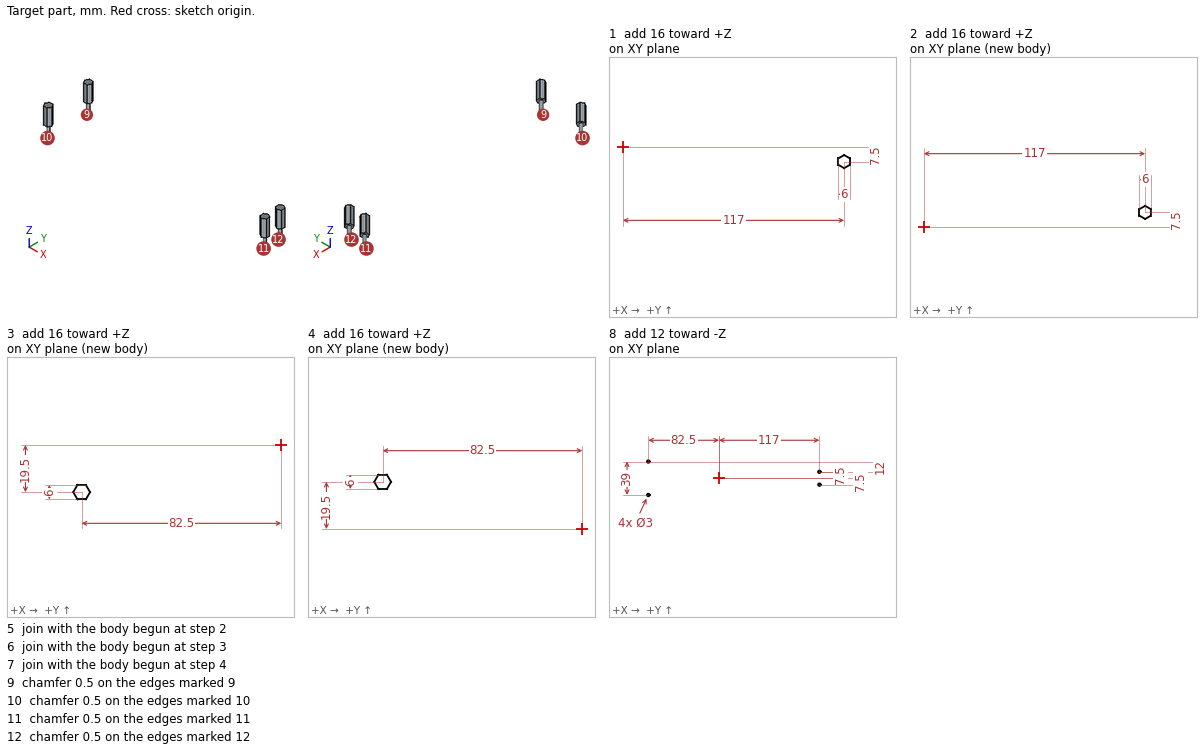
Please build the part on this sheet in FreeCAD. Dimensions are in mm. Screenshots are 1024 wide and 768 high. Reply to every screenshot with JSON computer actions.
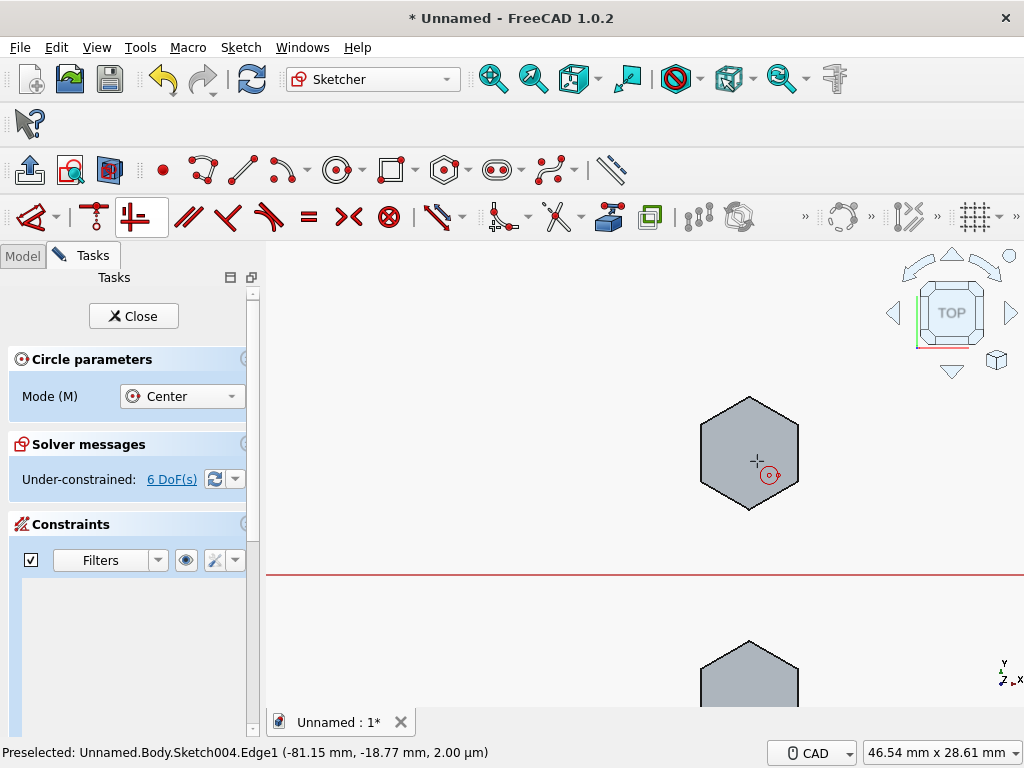
{"action": "scroll", "coordinate": [757, 461], "scroll_direction": "down", "scroll_amount": 11}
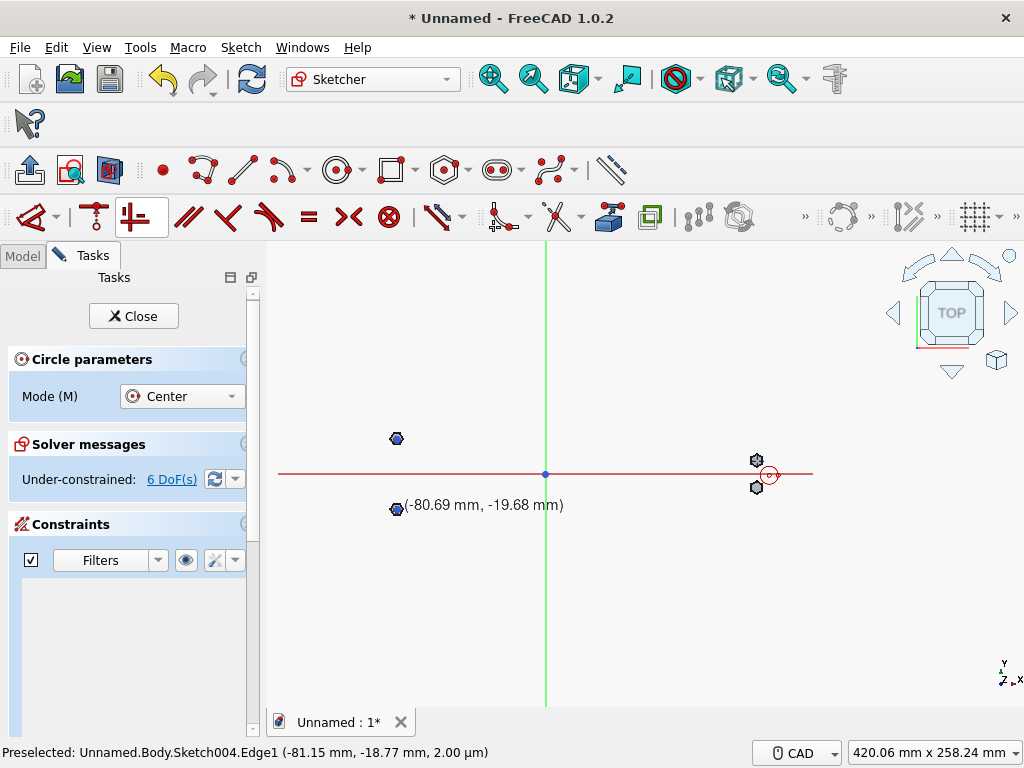
{"action": "left_click", "coordinate": [757, 461]}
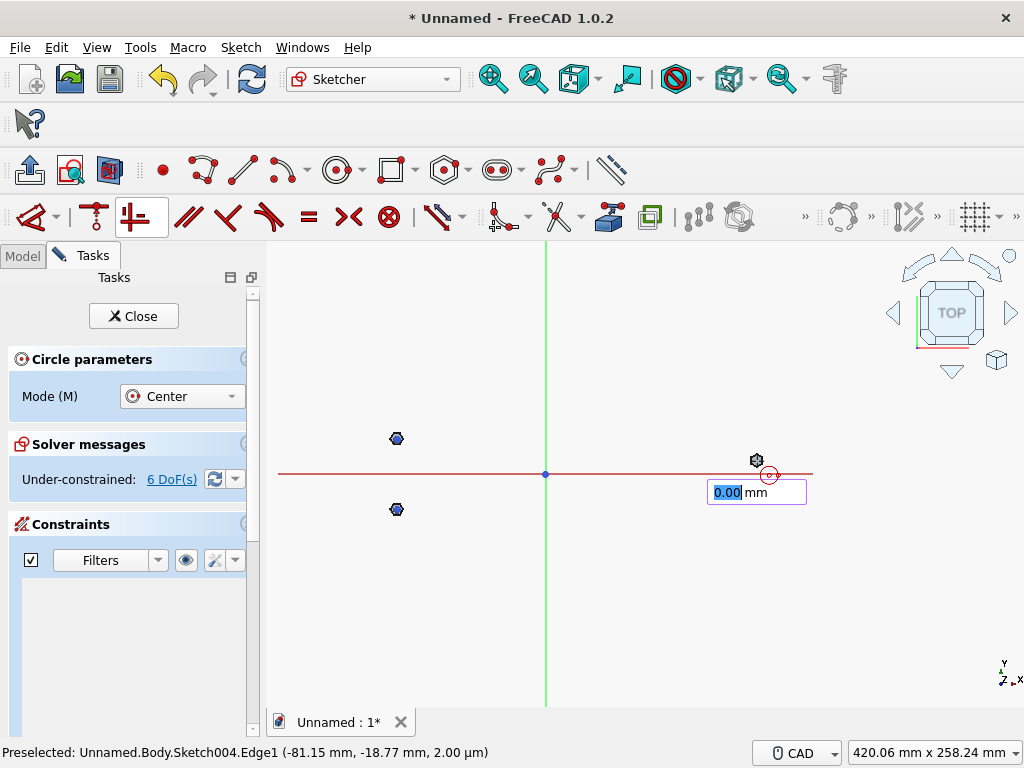
{"action": "scroll", "coordinate": [759, 459], "scroll_direction": "up", "scroll_amount": 9}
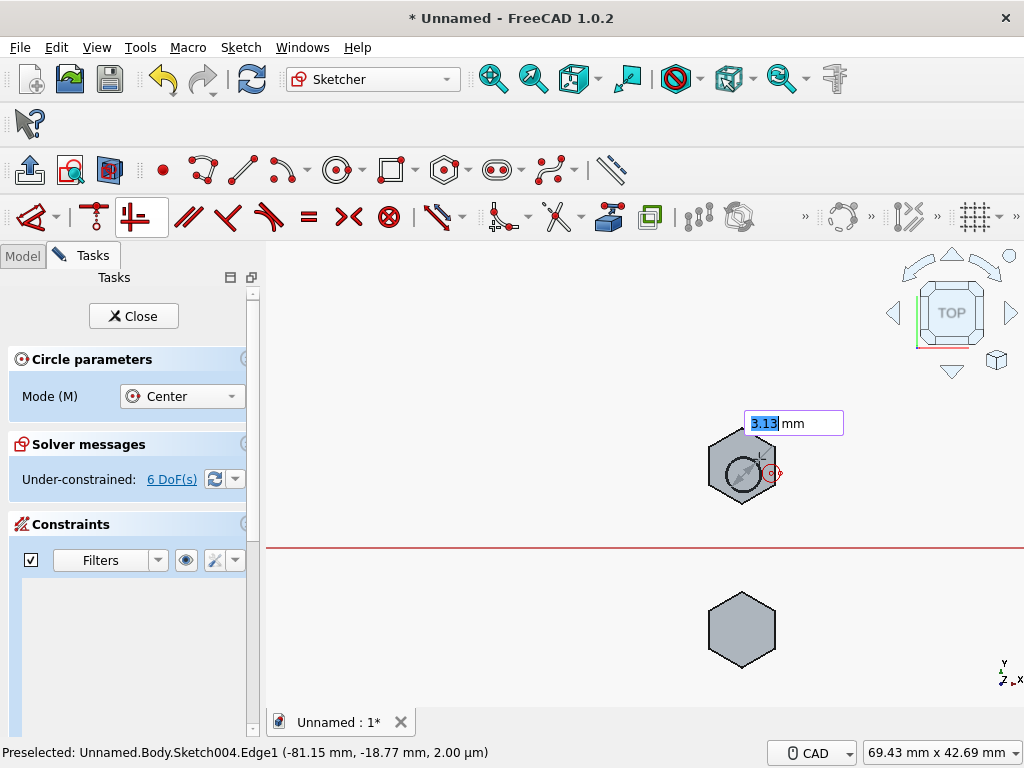
{"action": "left_click", "coordinate": [754, 454]}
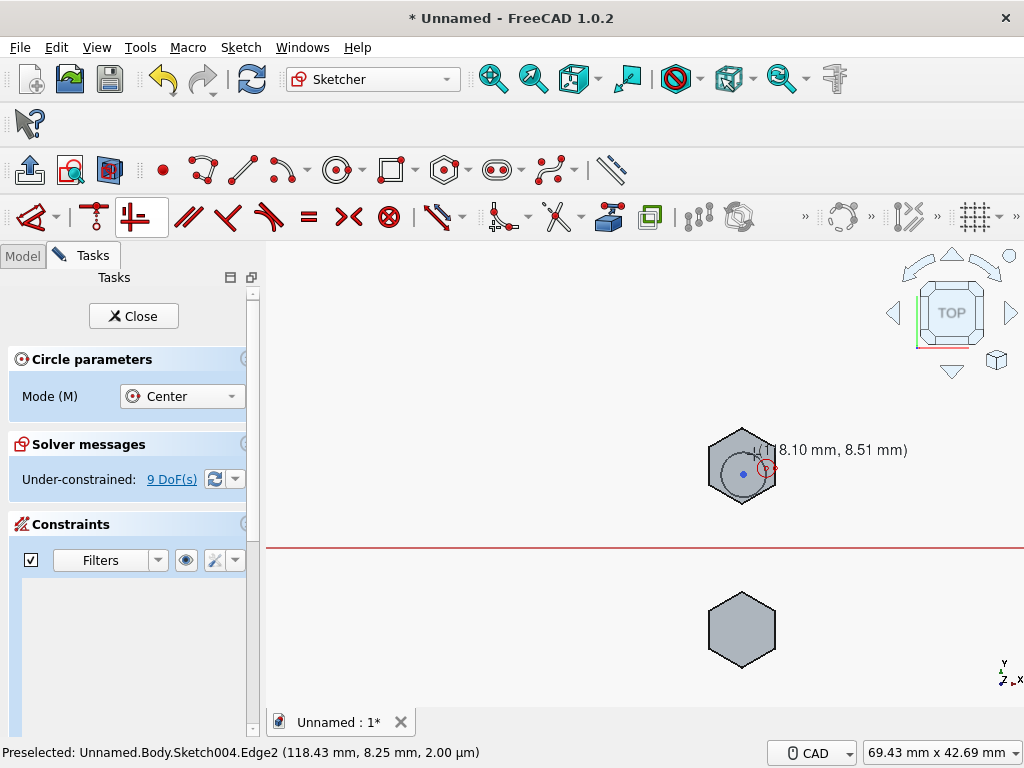
{"action": "scroll", "coordinate": [742, 630], "scroll_direction": "up", "scroll_amount": 2}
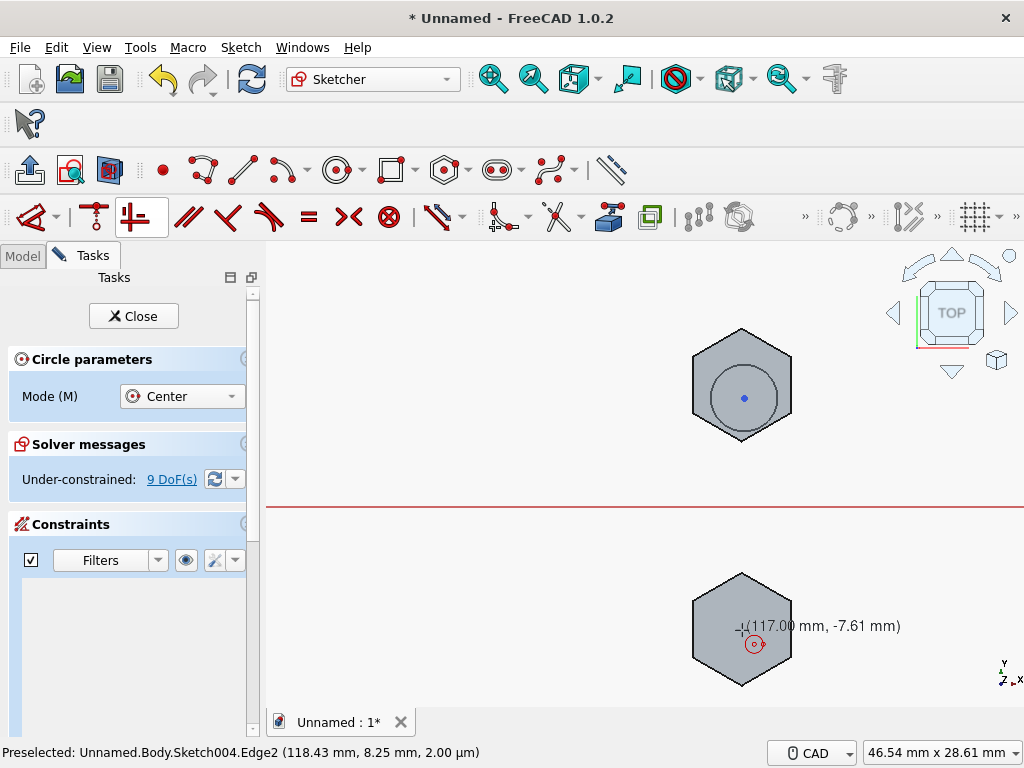
{"action": "scroll", "coordinate": [758, 470], "scroll_direction": "down", "scroll_amount": 11}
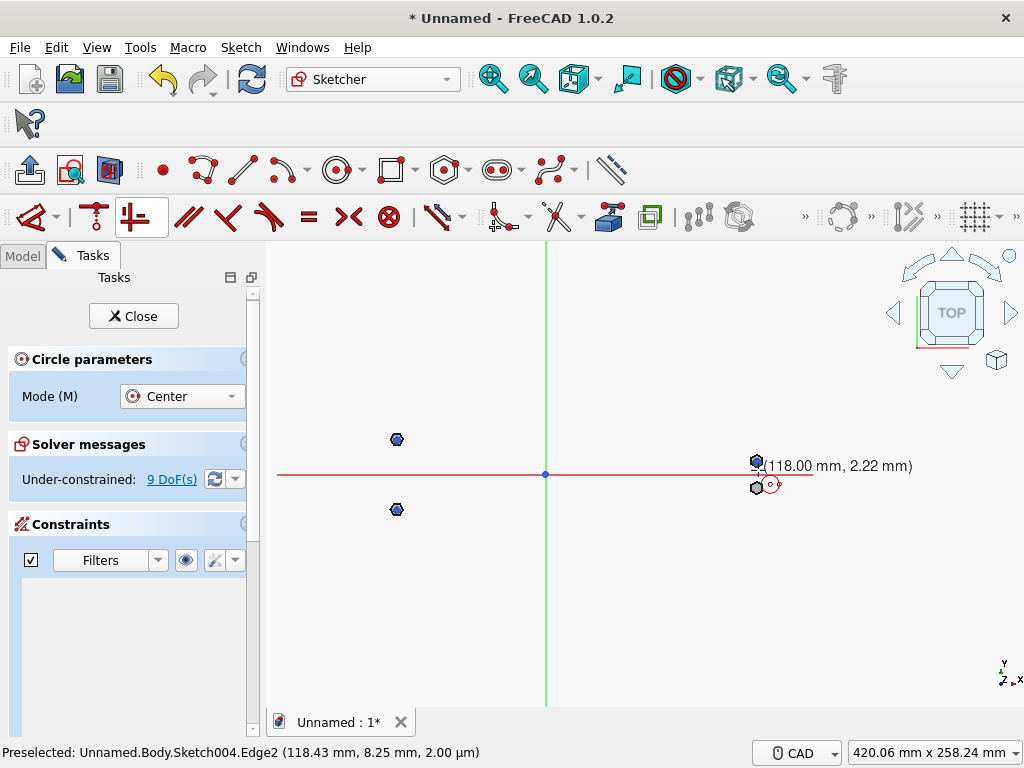
{"action": "left_click", "coordinate": [757, 488]}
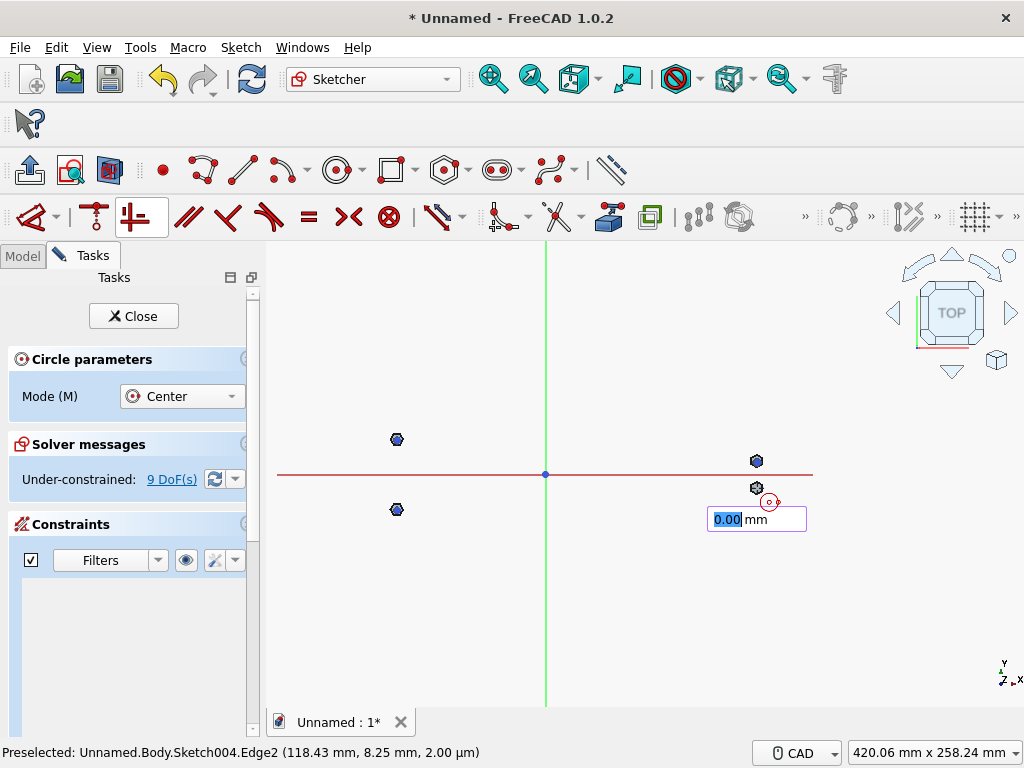
{"action": "scroll", "coordinate": [759, 490], "scroll_direction": "up", "scroll_amount": 9}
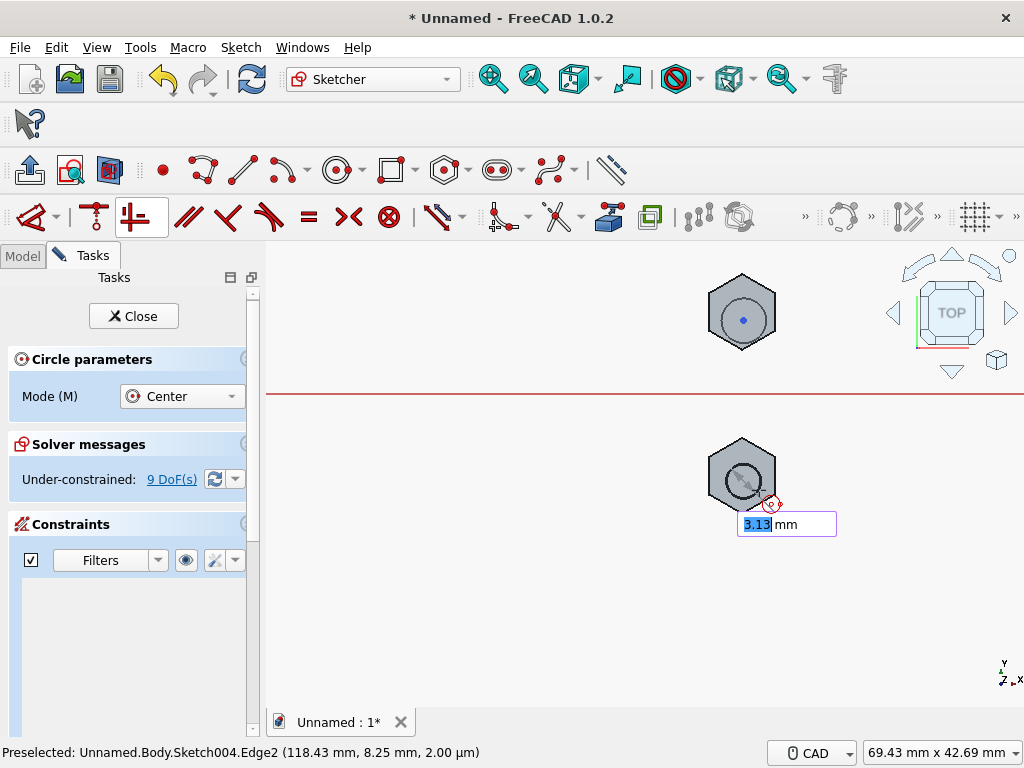
{"action": "left_click", "coordinate": [754, 487]}
{"action": "key", "text": "Escape"}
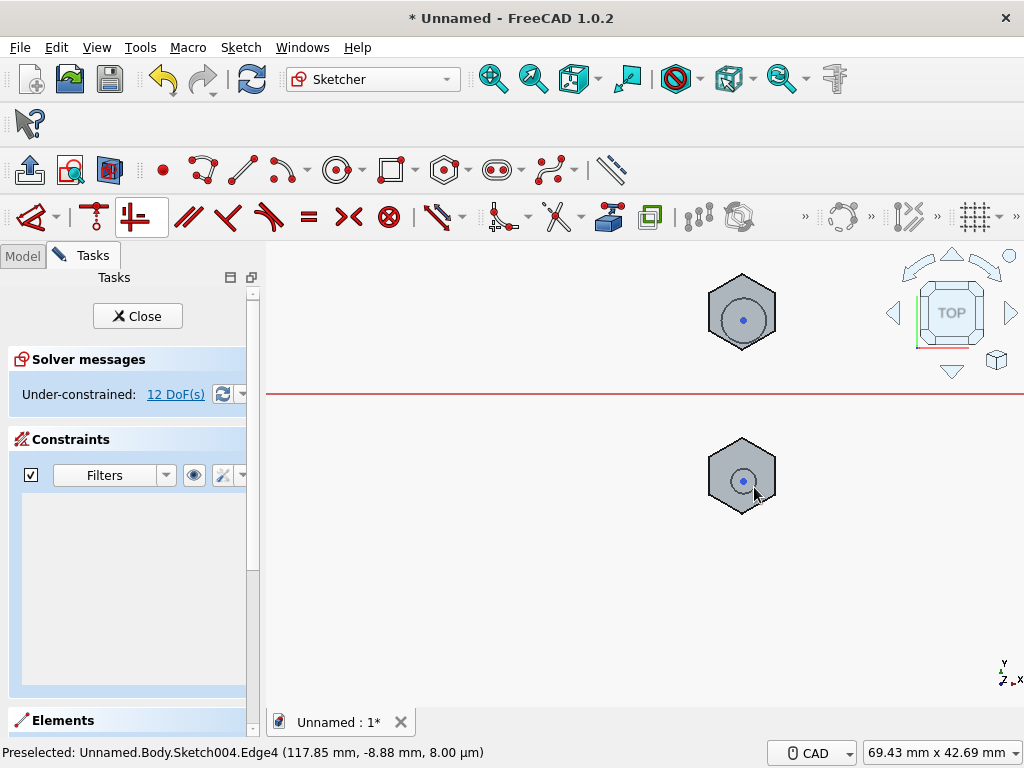
{"action": "scroll", "coordinate": [759, 490], "scroll_direction": "down", "scroll_amount": 9}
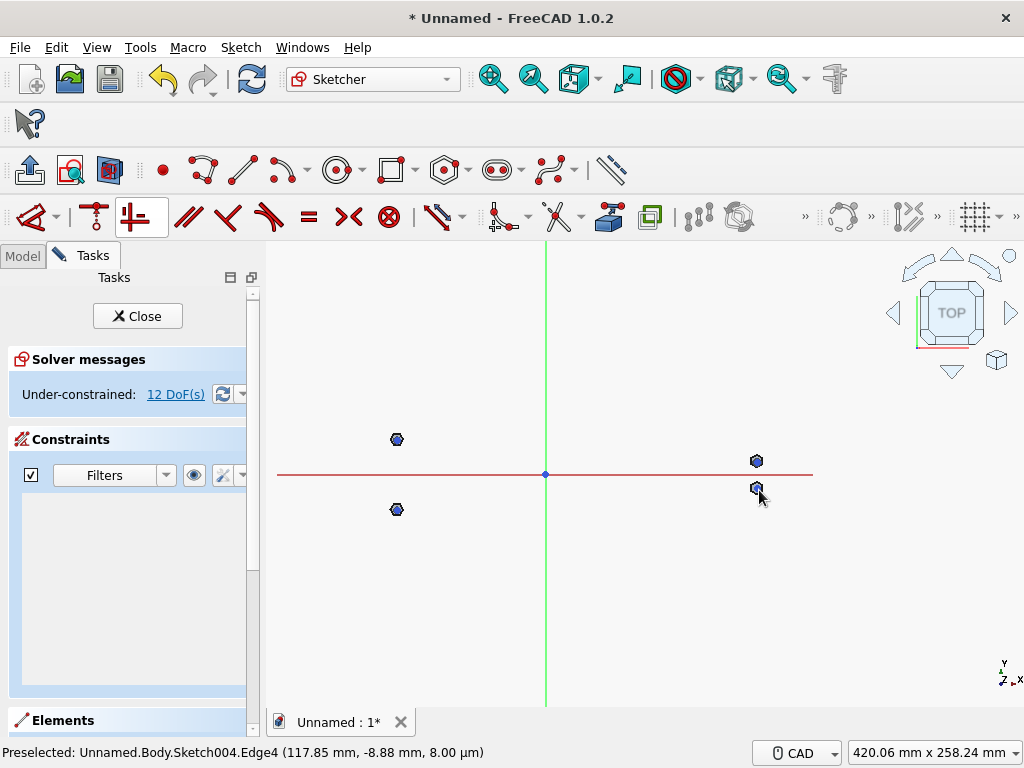
{"action": "scroll", "coordinate": [399, 438], "scroll_direction": "up", "scroll_amount": 8}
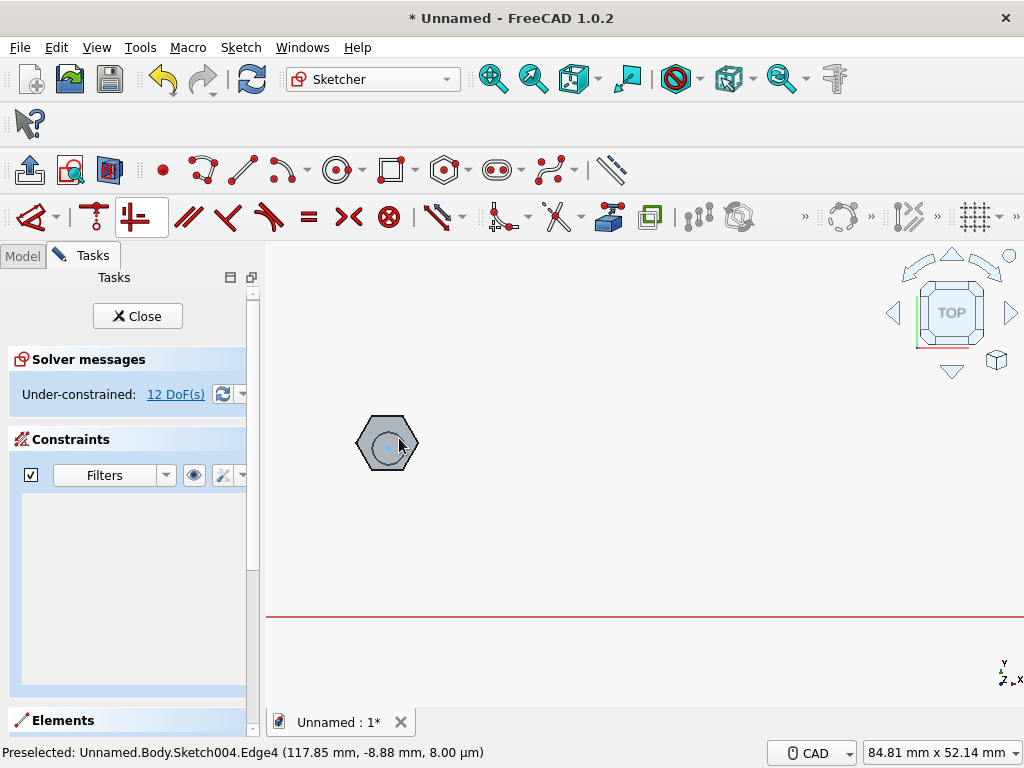
{"action": "left_click", "coordinate": [400, 437]}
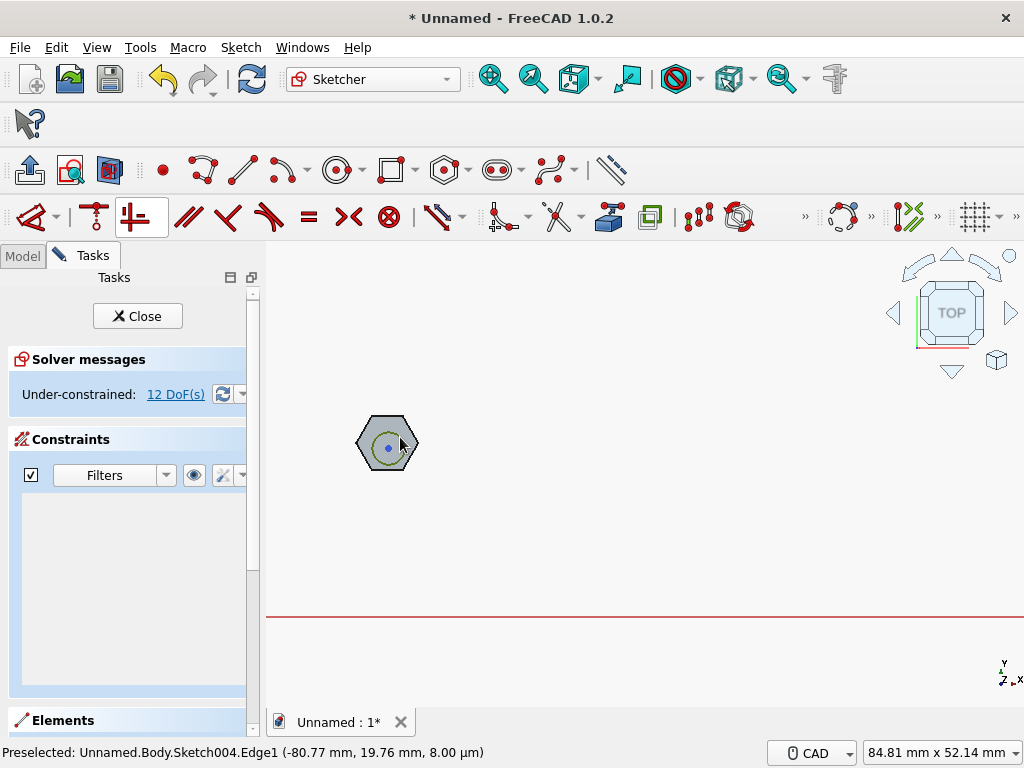
{"action": "scroll", "coordinate": [399, 438], "scroll_direction": "down", "scroll_amount": 8}